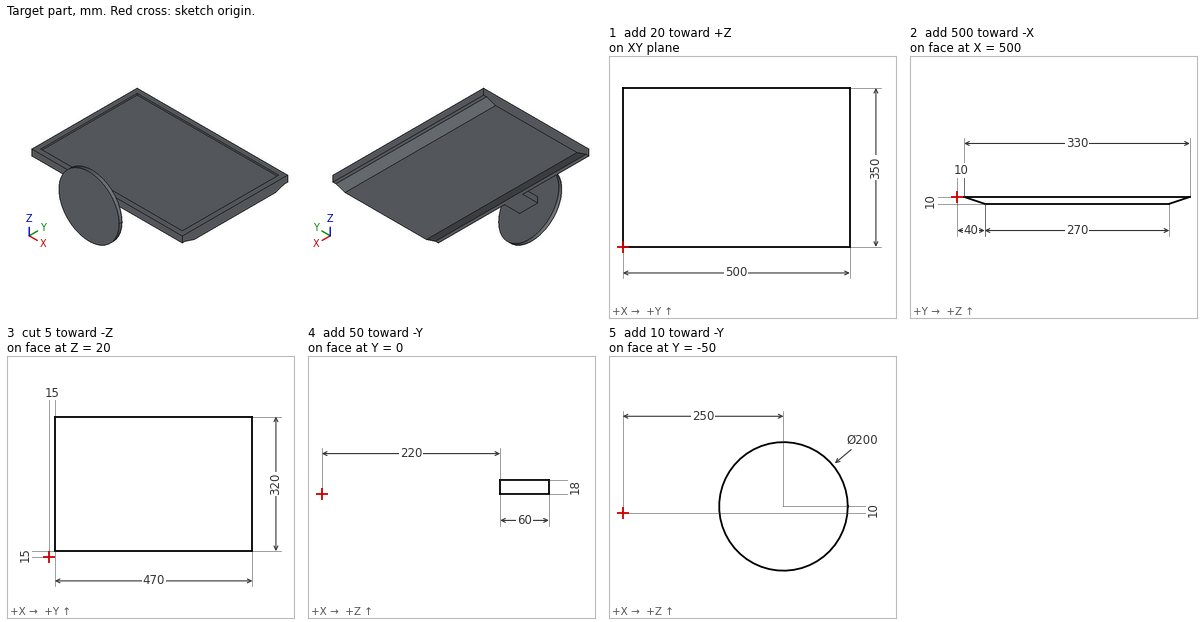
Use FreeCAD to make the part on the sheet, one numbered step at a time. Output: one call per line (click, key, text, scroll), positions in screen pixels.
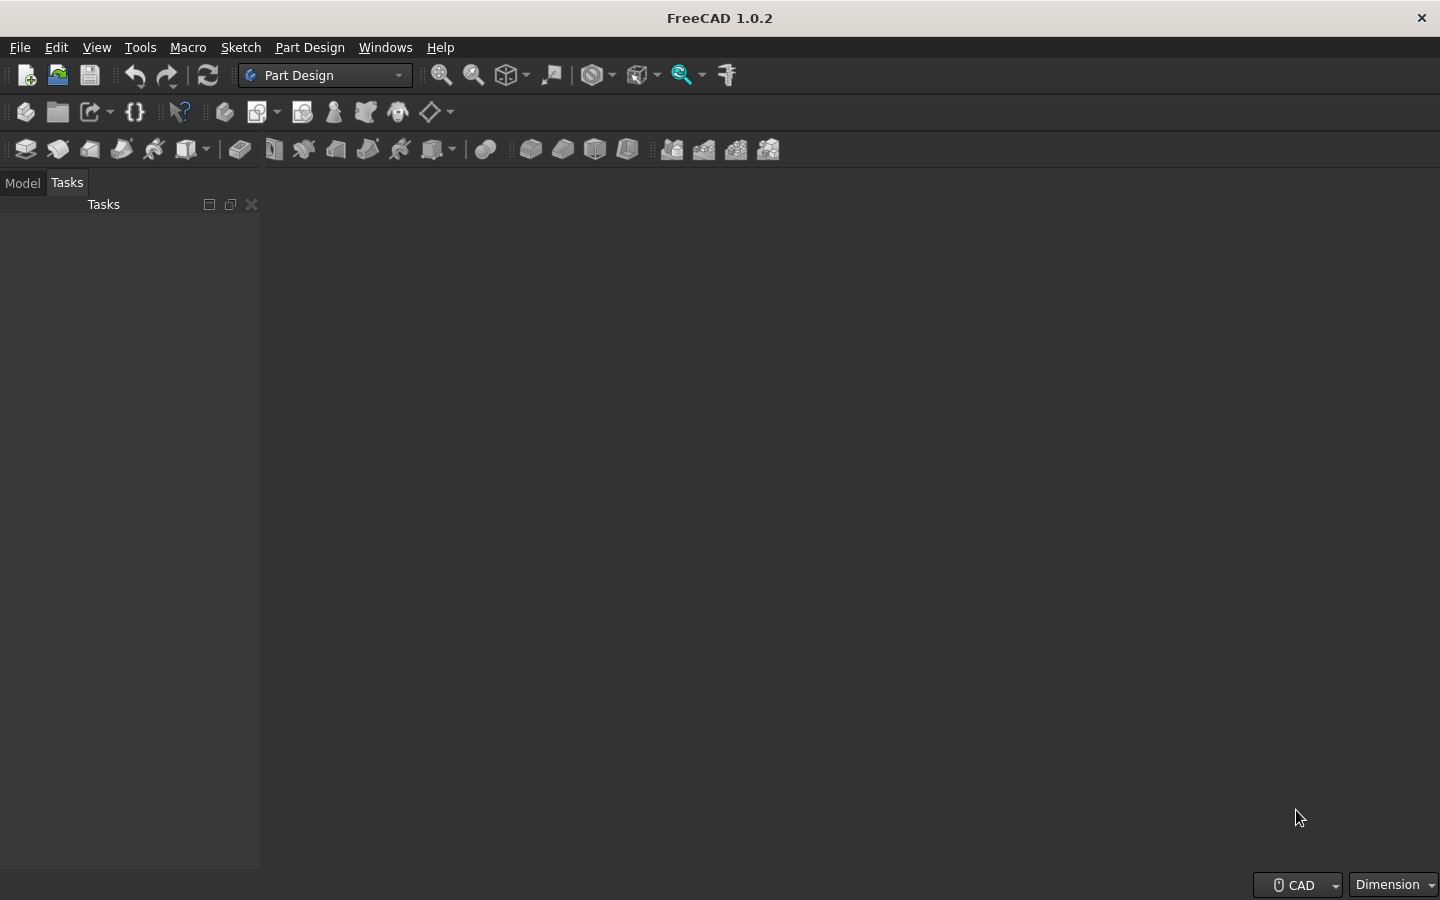
key(ctrl+n)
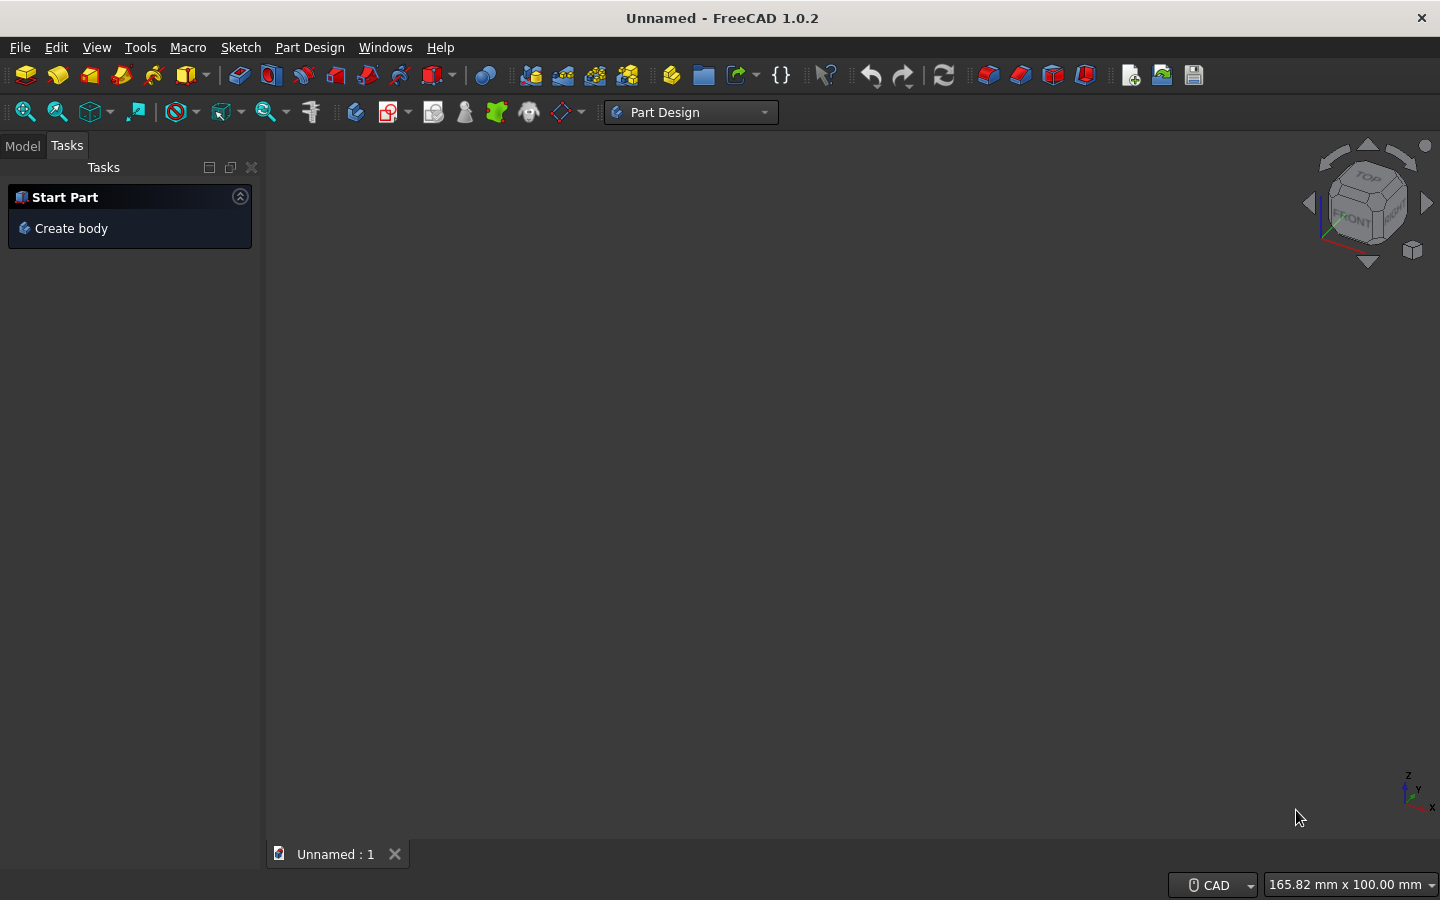
click(388, 112)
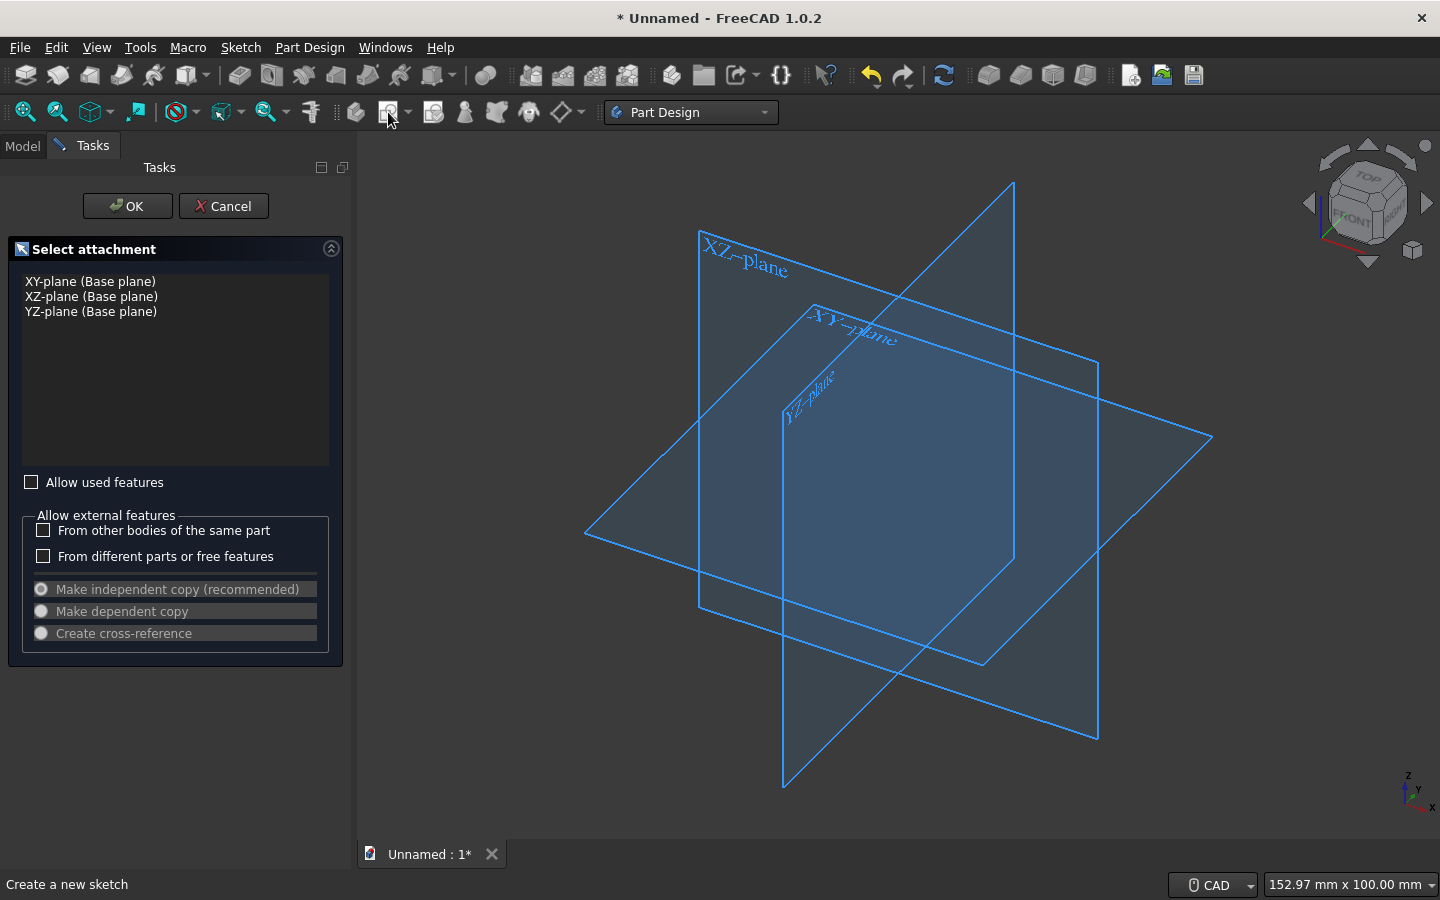
click(82, 282)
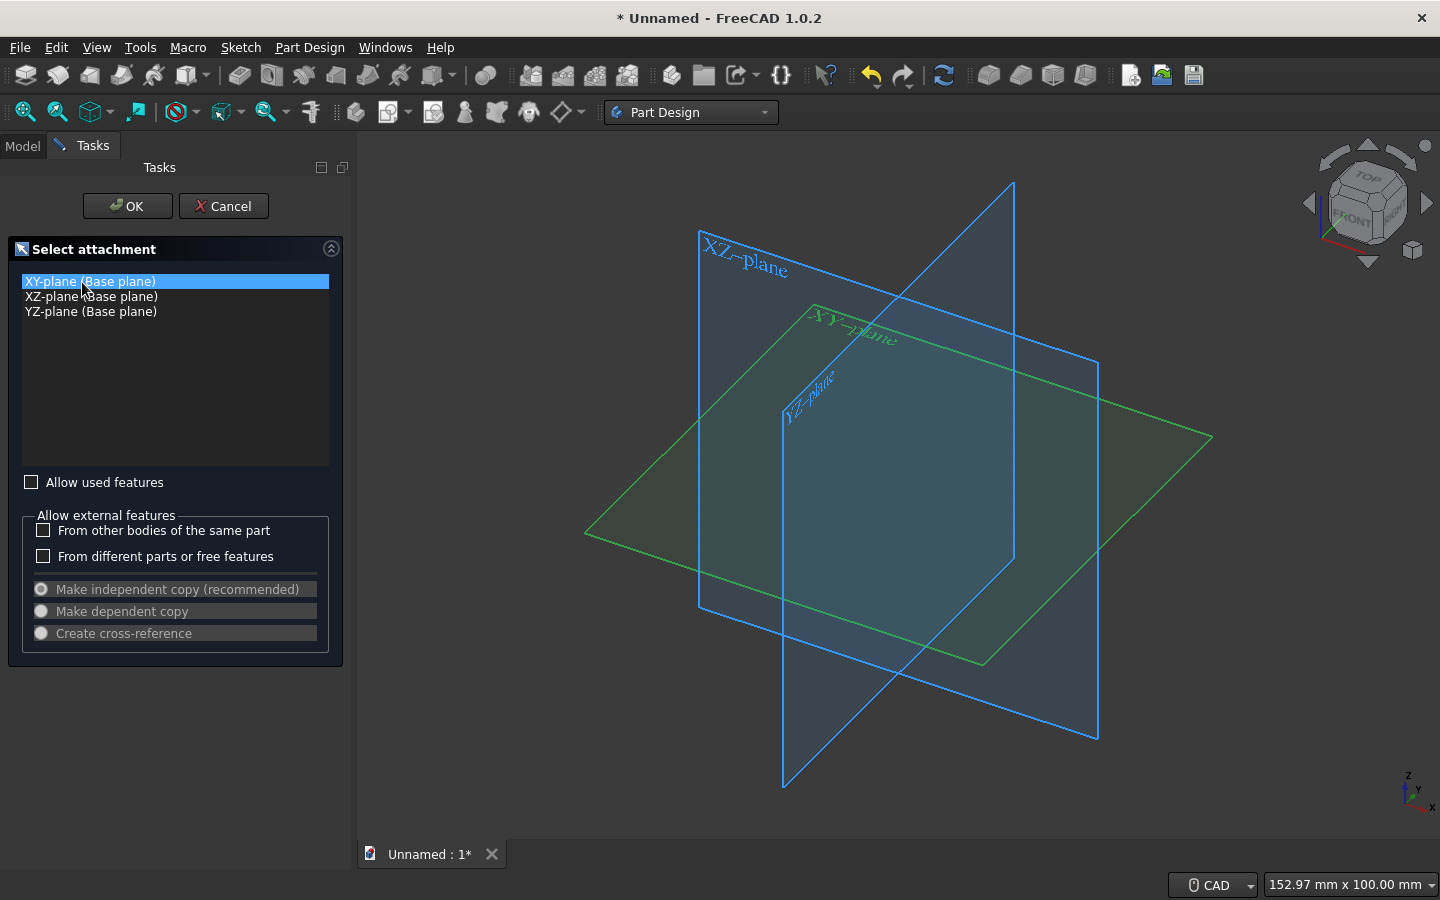
click(128, 206)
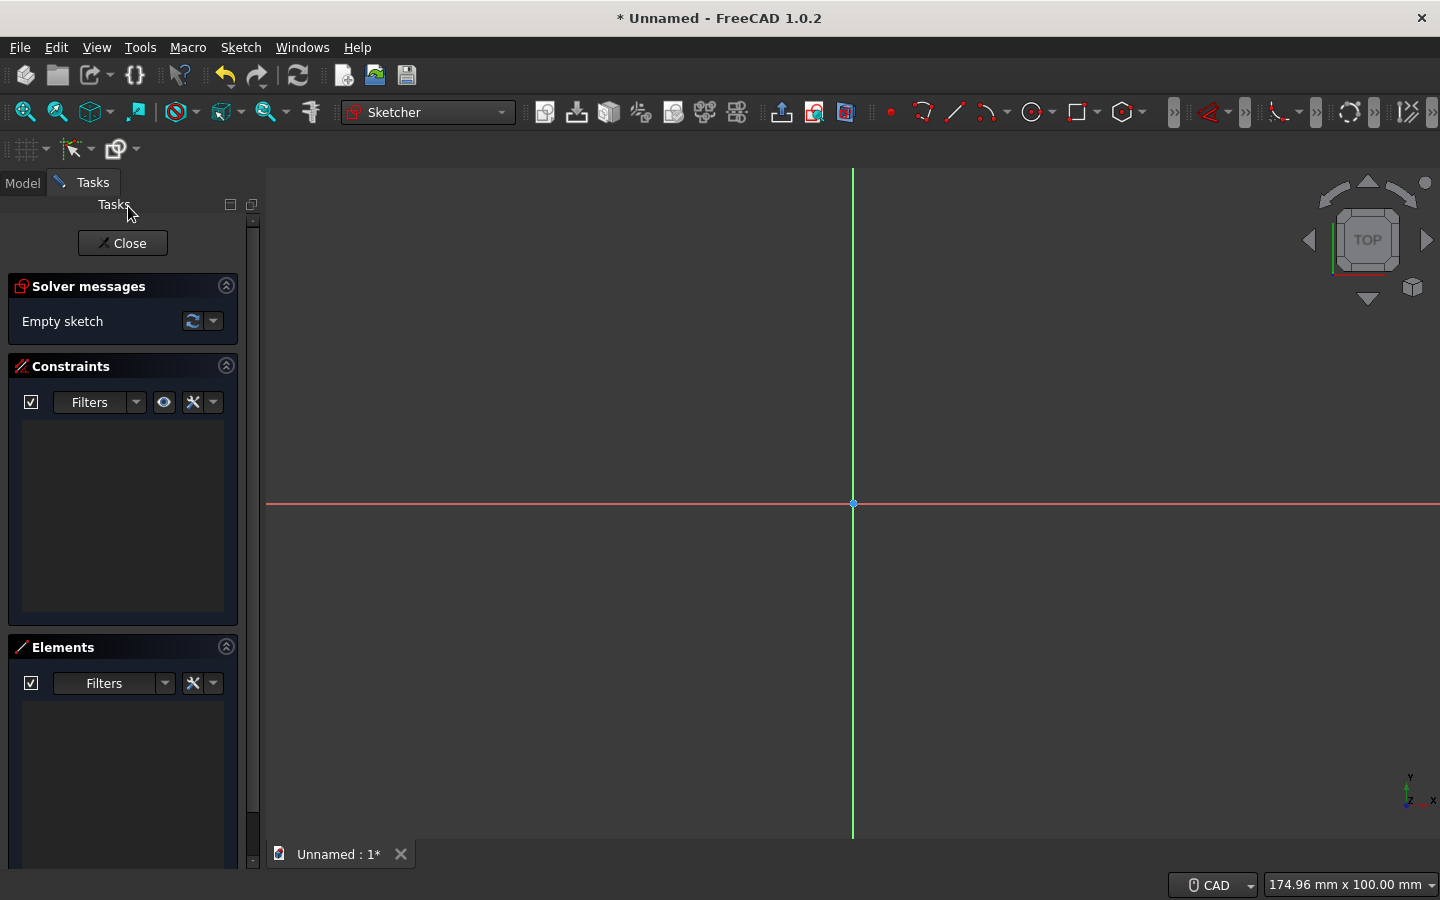
scroll(343, 801, down, 8)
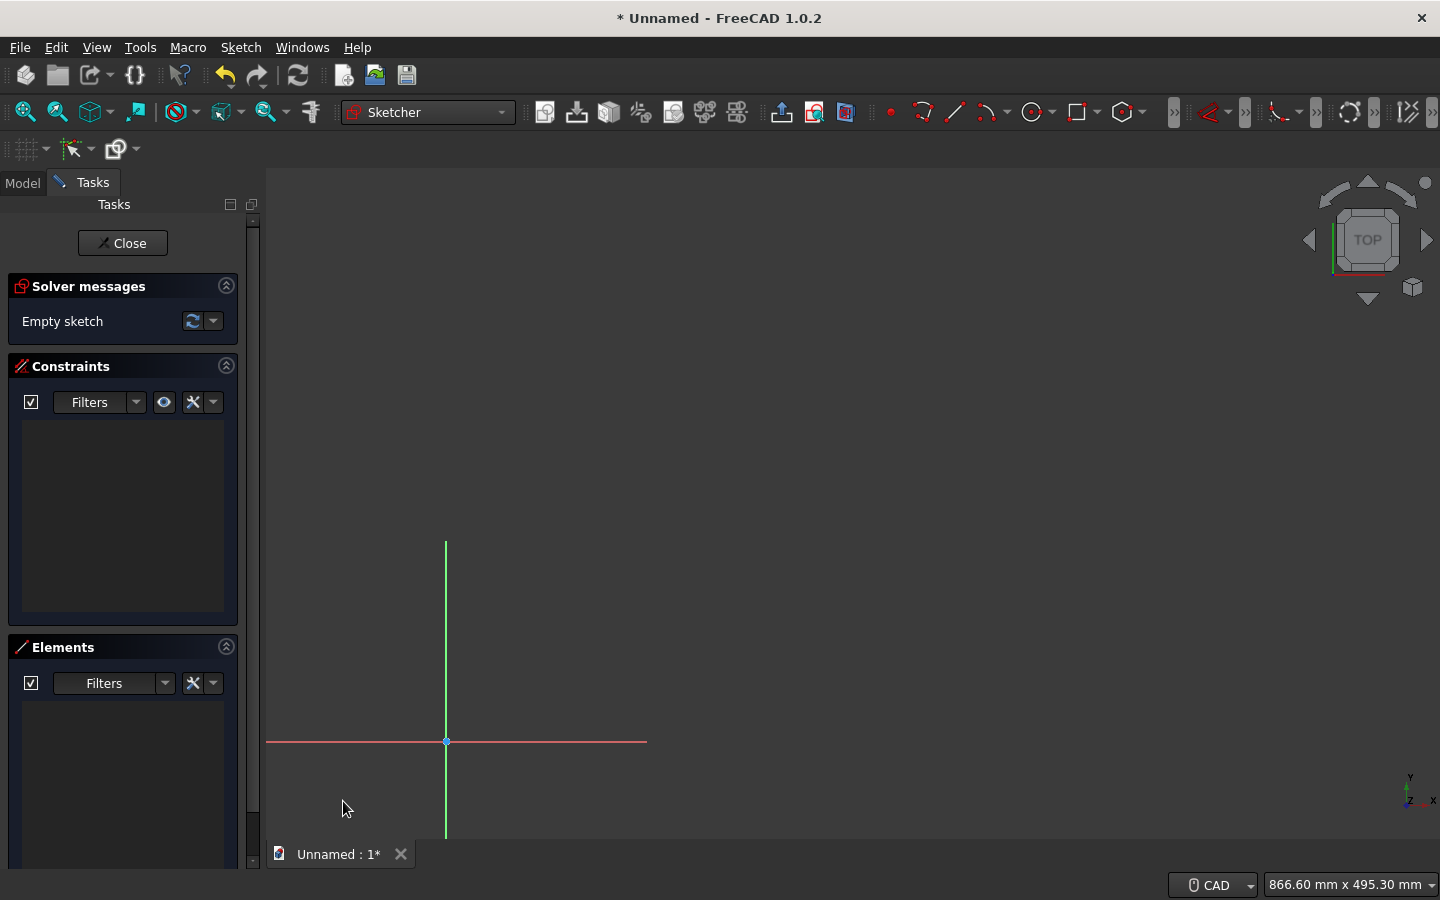
key(g)
key(r)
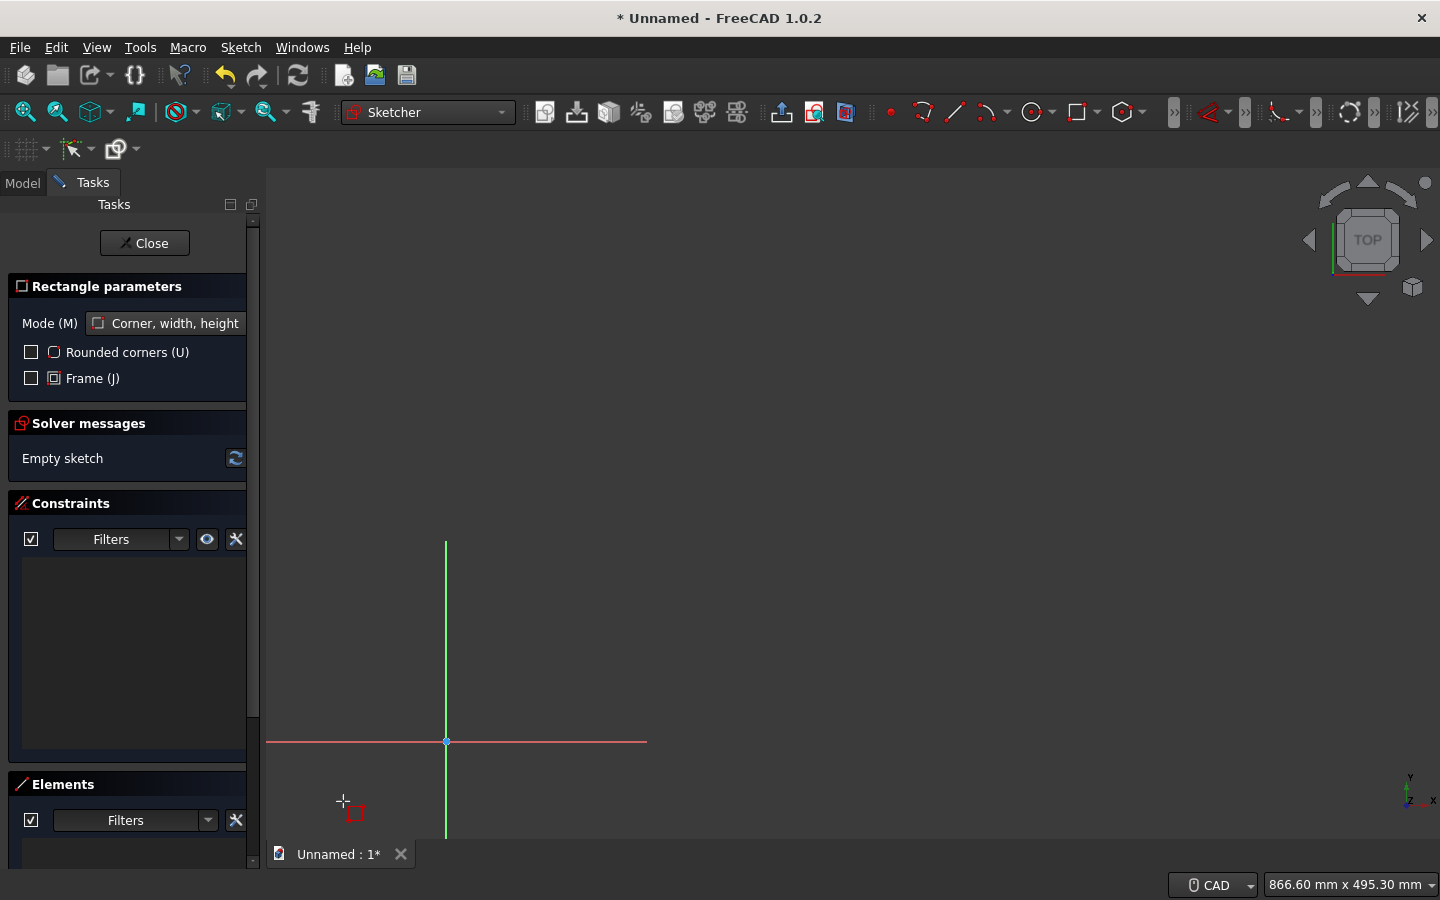
click(446, 742)
move(1123, 268)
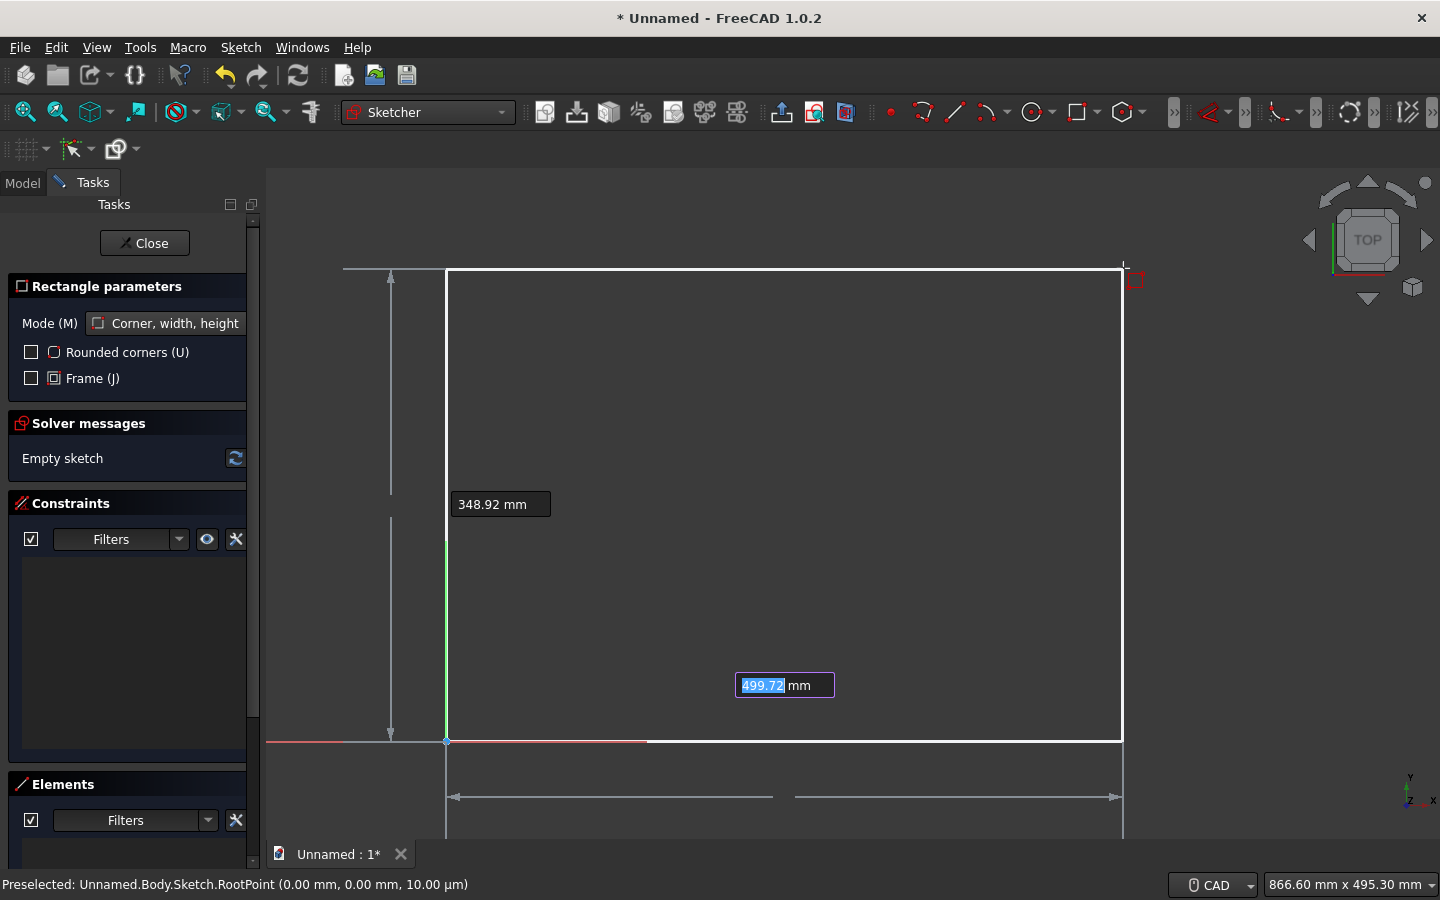
text(500)
key(Tab)
text(350)
key(Return)
key(Escape)